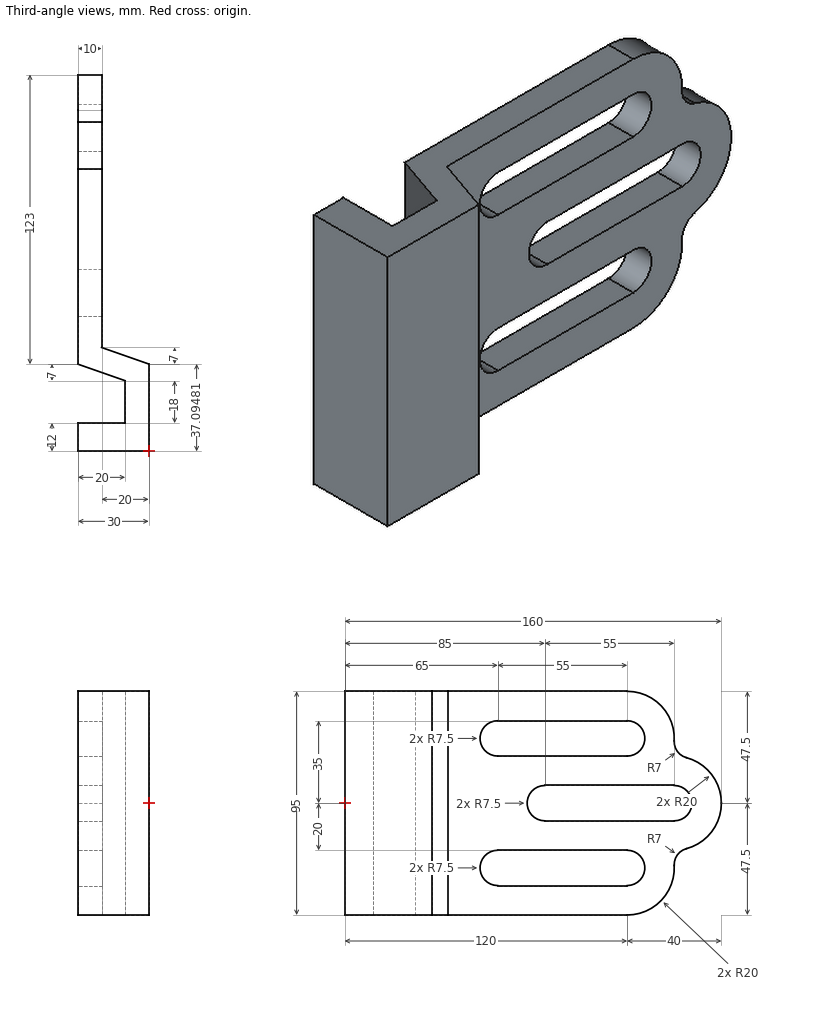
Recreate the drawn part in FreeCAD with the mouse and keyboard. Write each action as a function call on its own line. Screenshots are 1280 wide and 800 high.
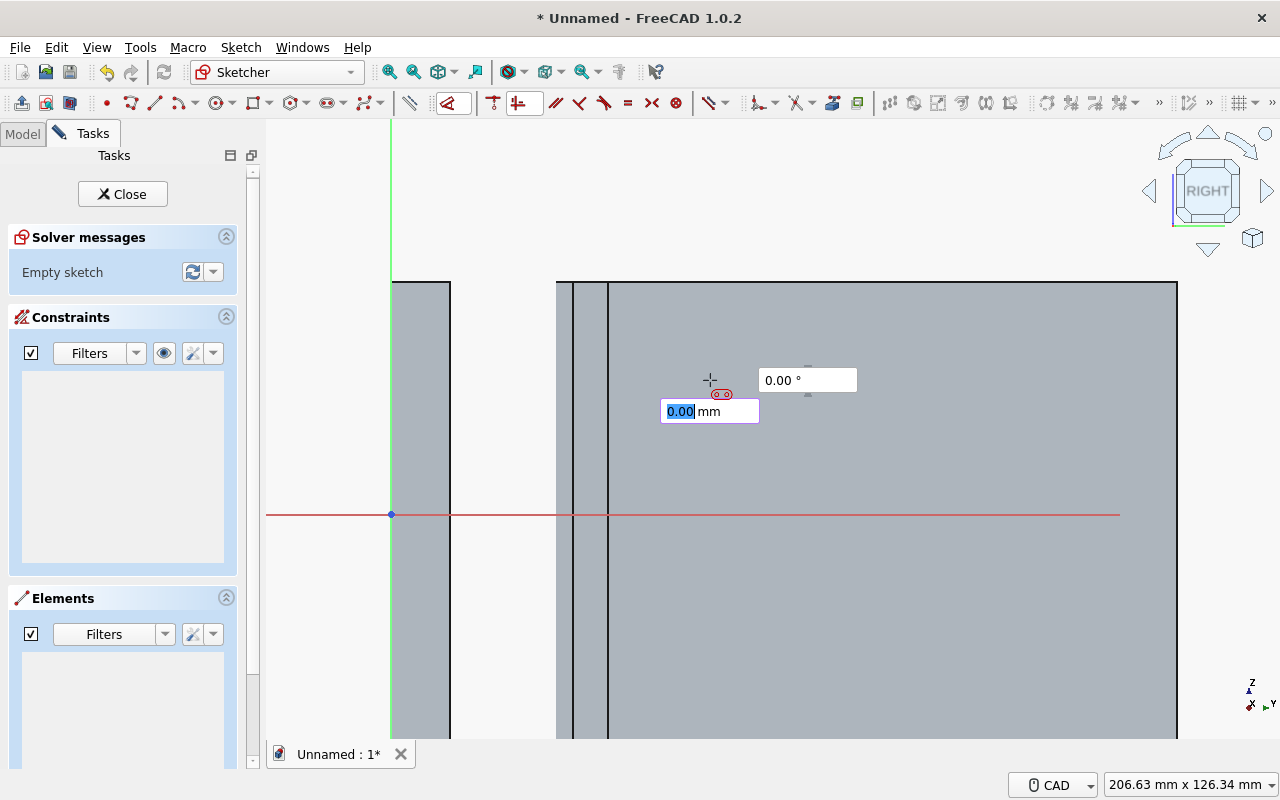
click(980, 380)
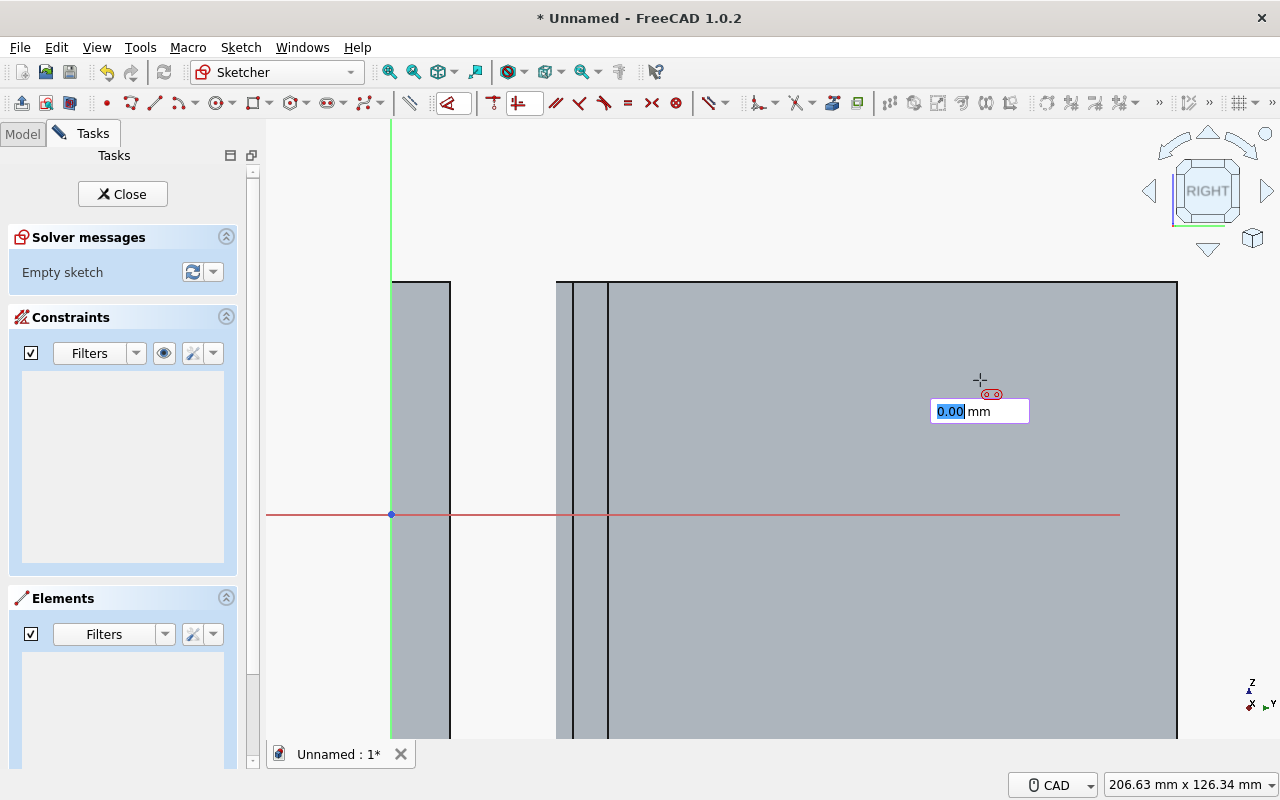
click(845, 343)
key(Escape)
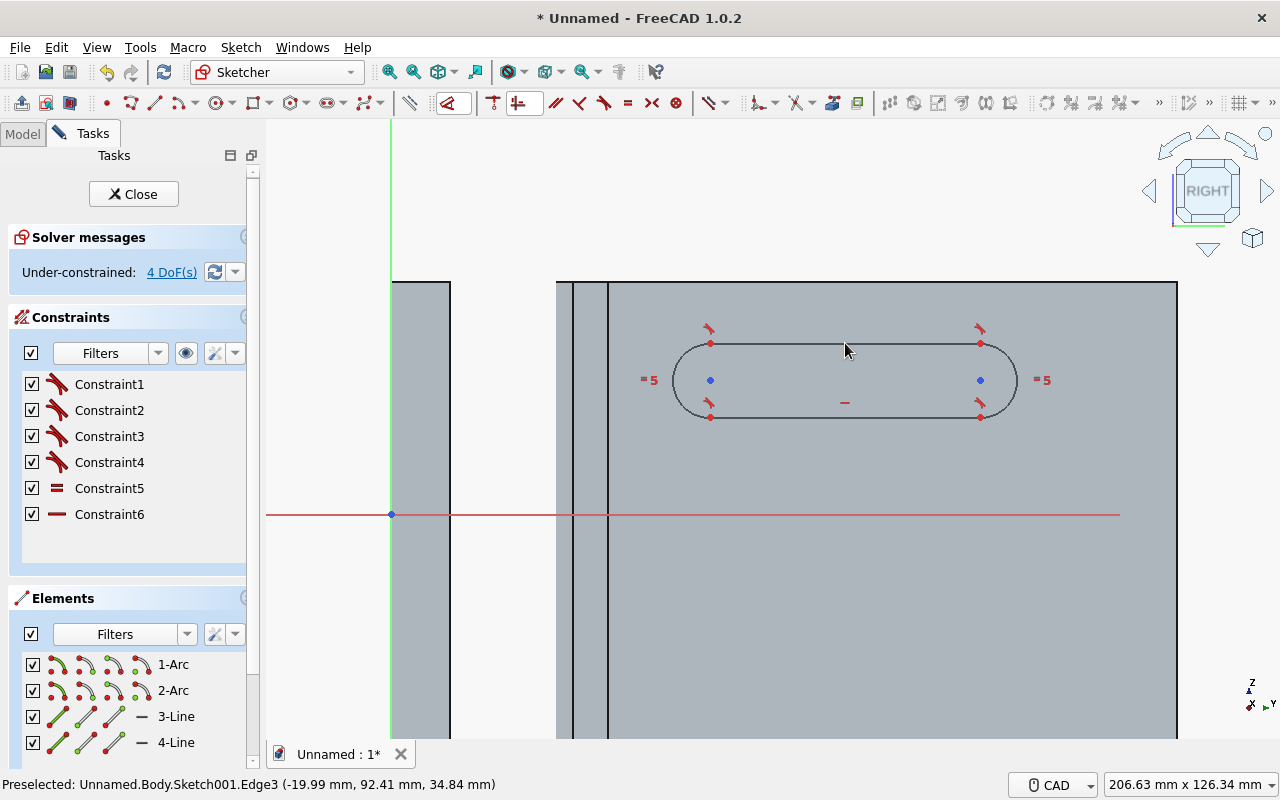
click(448, 104)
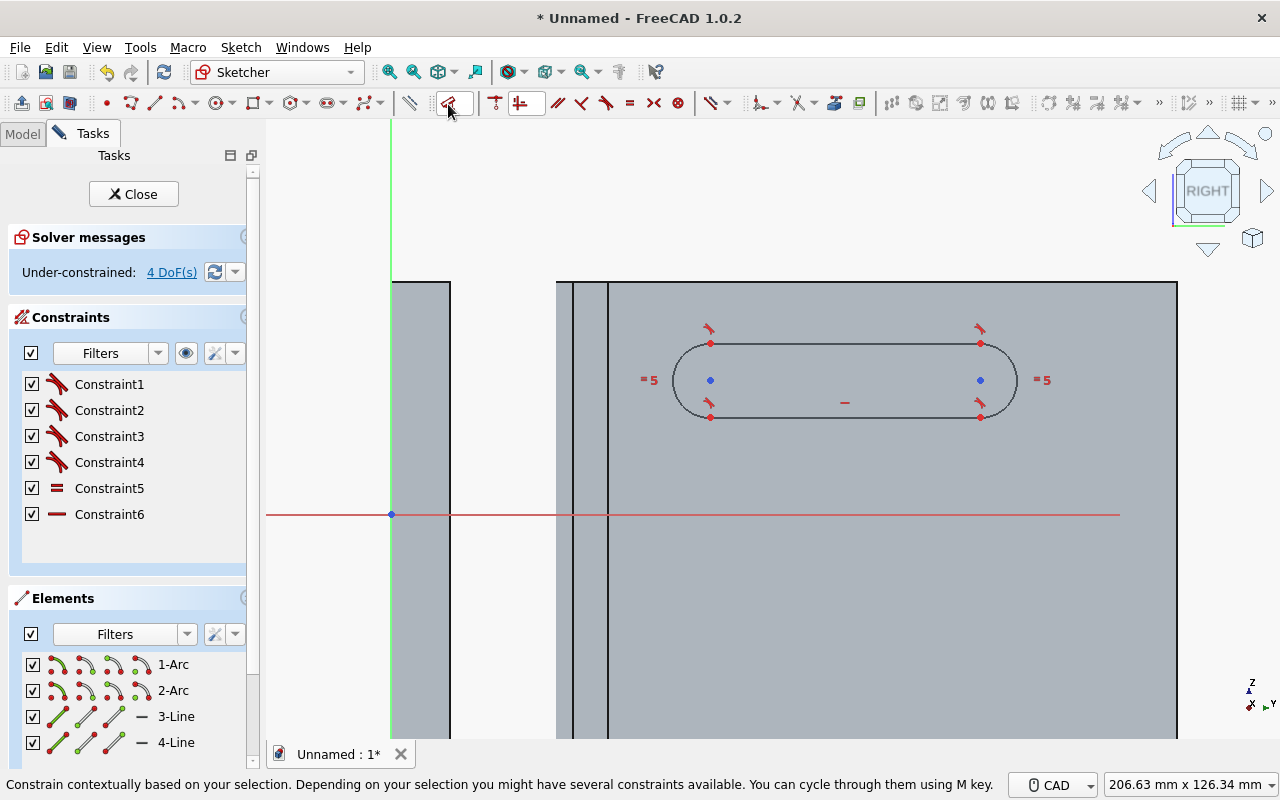
click(680, 359)
click(654, 340)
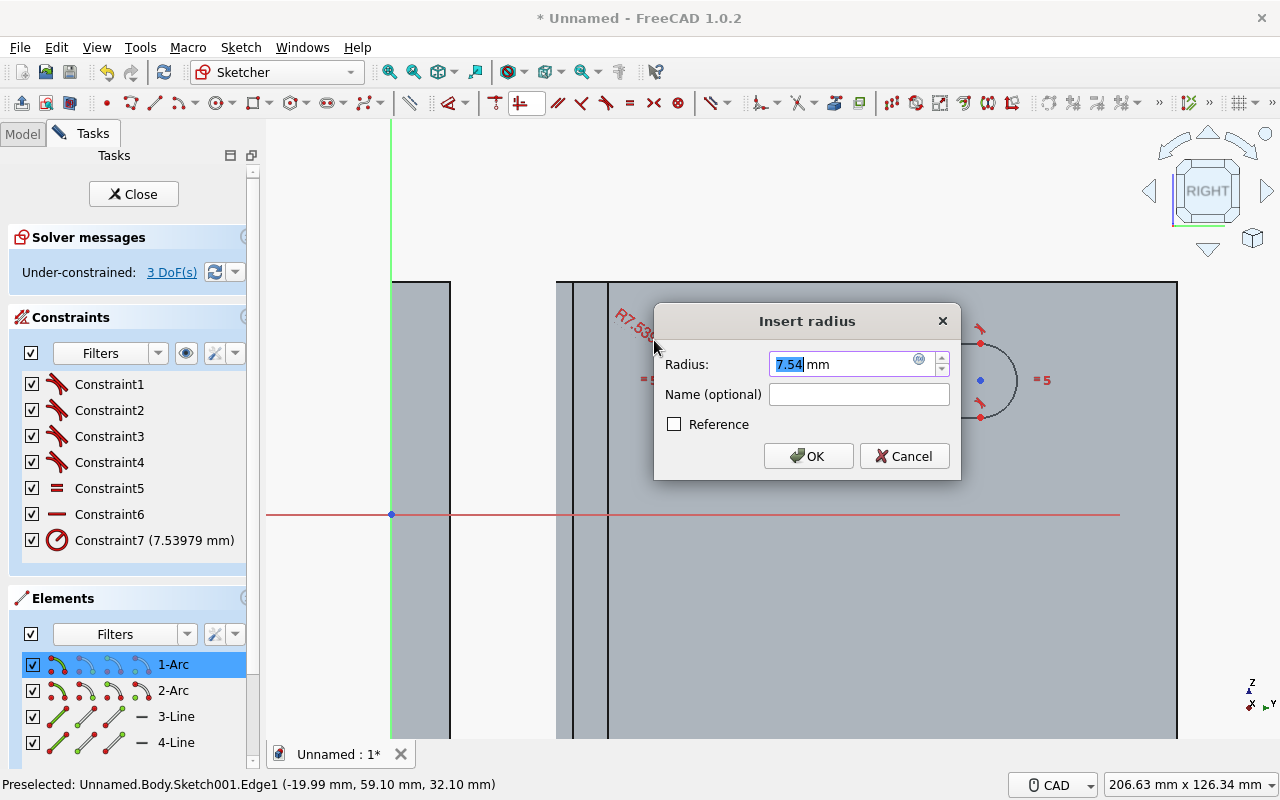
text(7.5)
key(Return)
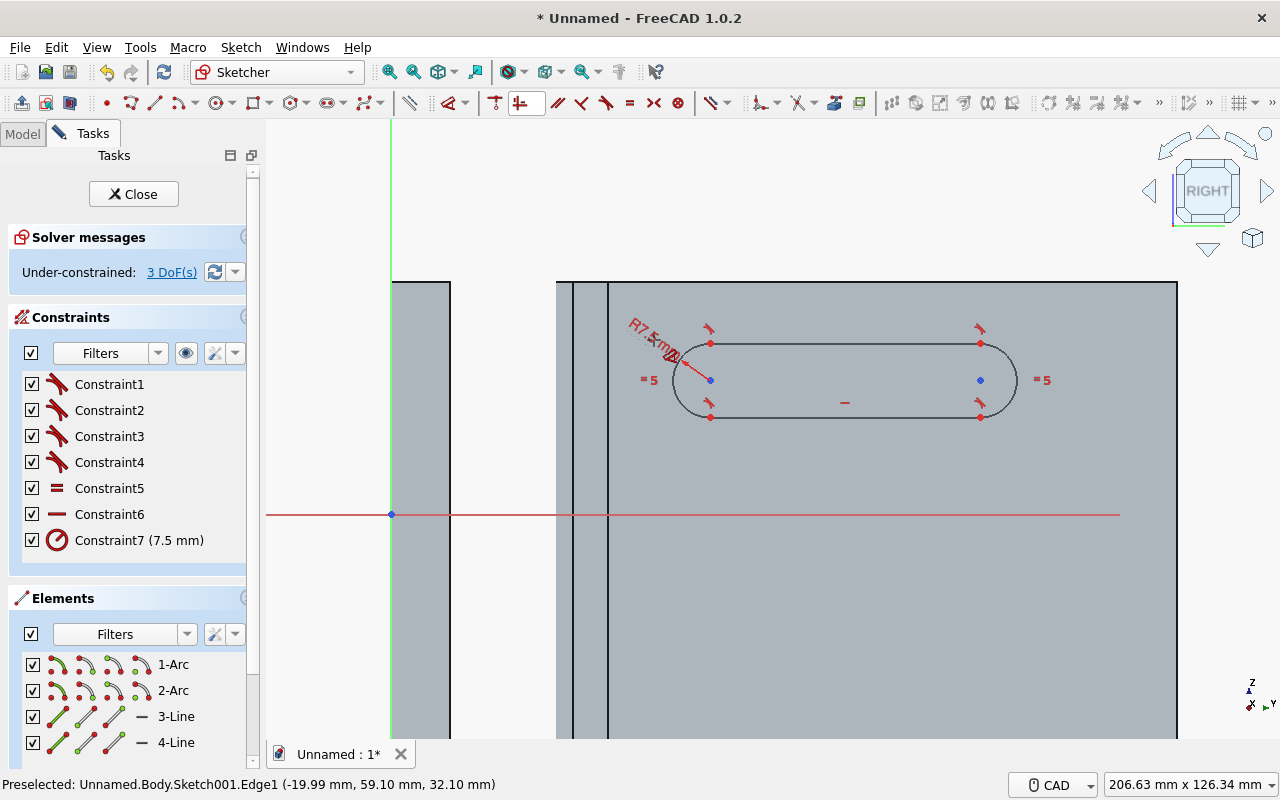
click(791, 344)
click(845, 310)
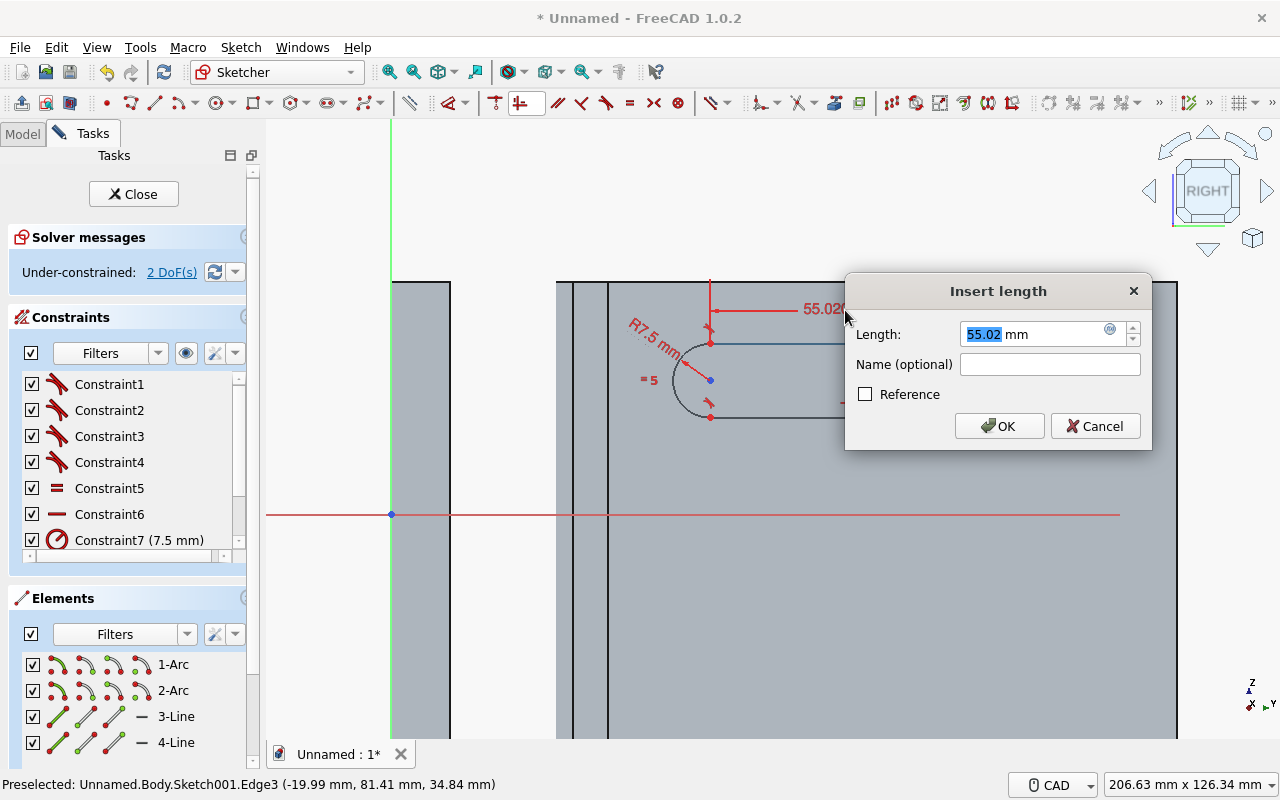
text(55)
key(Return)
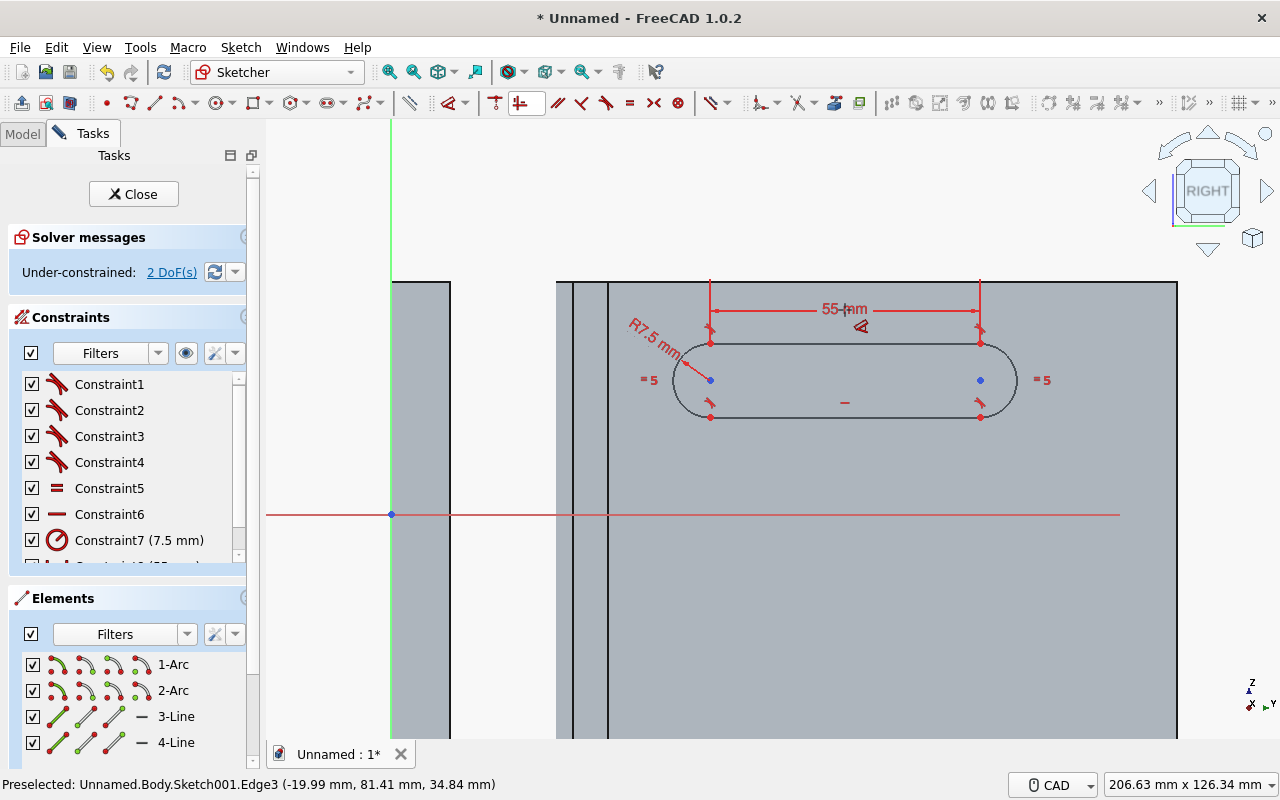
click(710, 344)
click(551, 549)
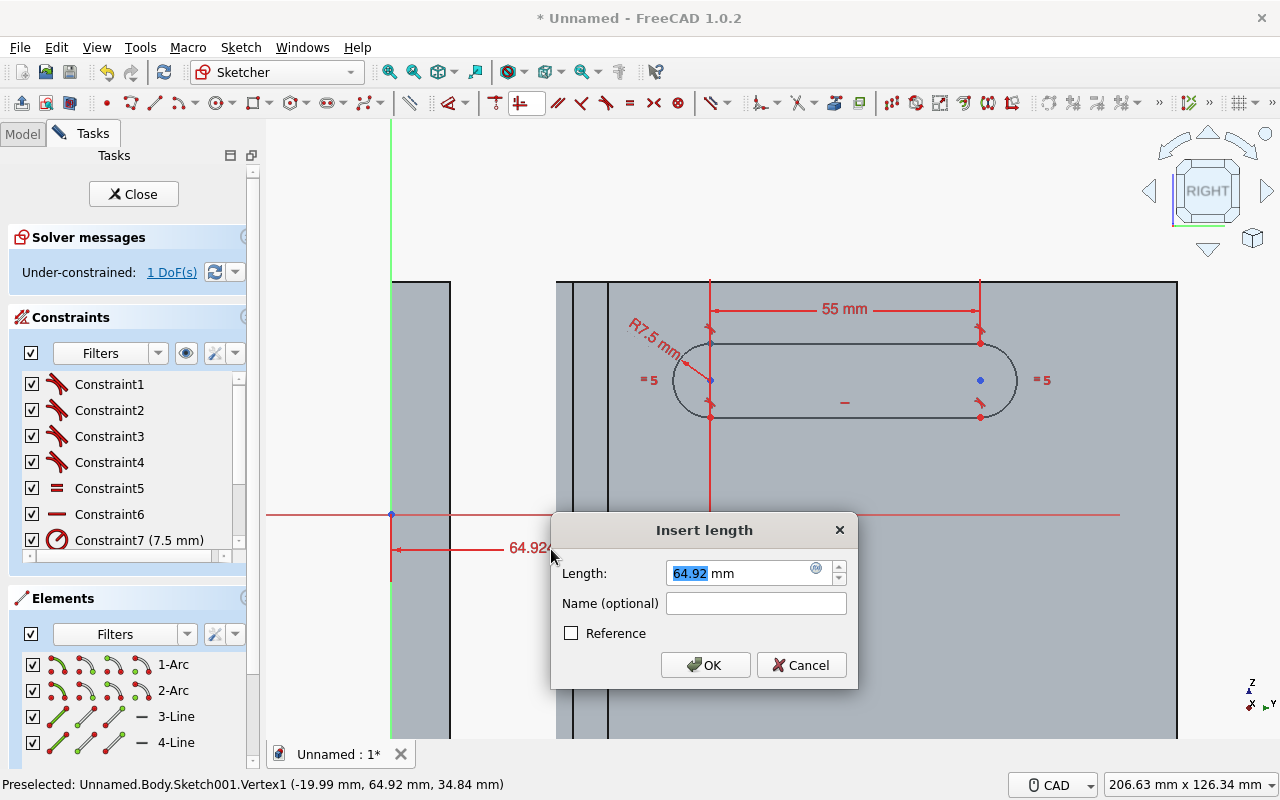
text(65)
key(Return)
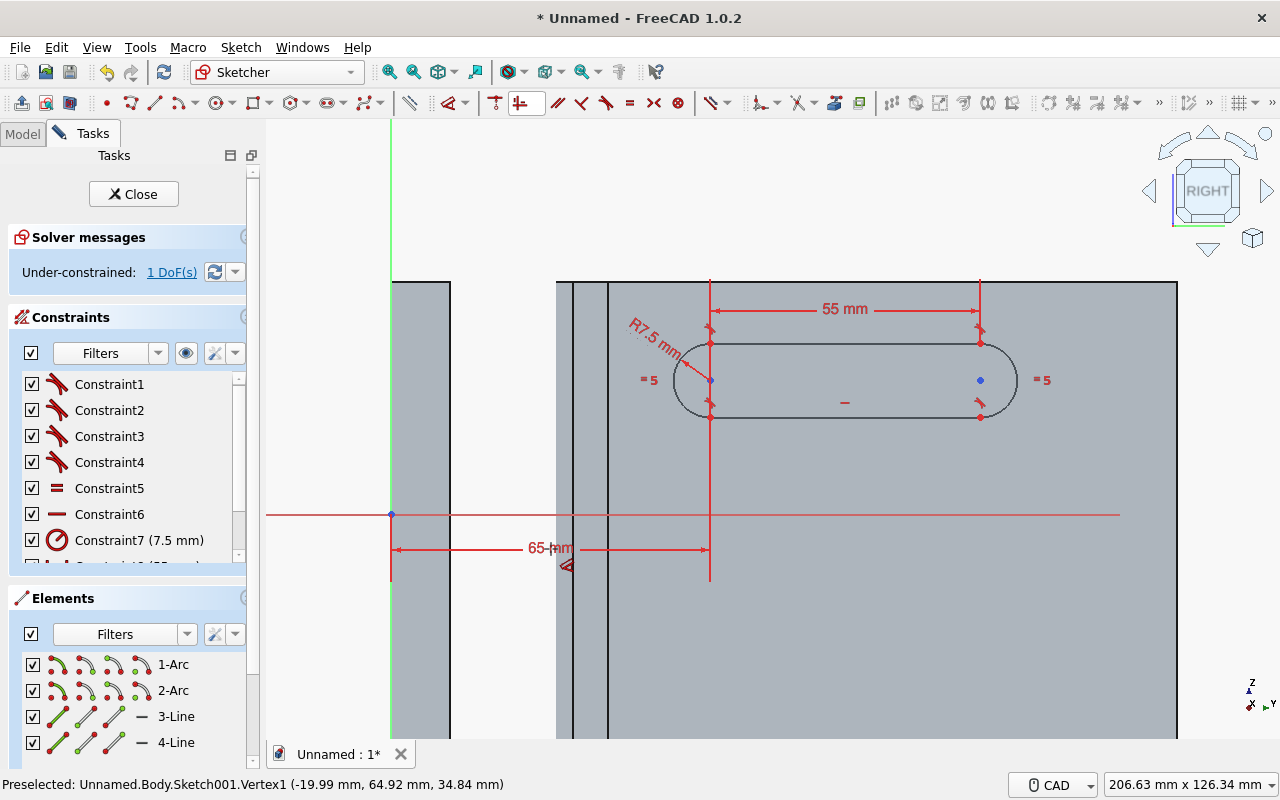
click(710, 344)
click(357, 429)